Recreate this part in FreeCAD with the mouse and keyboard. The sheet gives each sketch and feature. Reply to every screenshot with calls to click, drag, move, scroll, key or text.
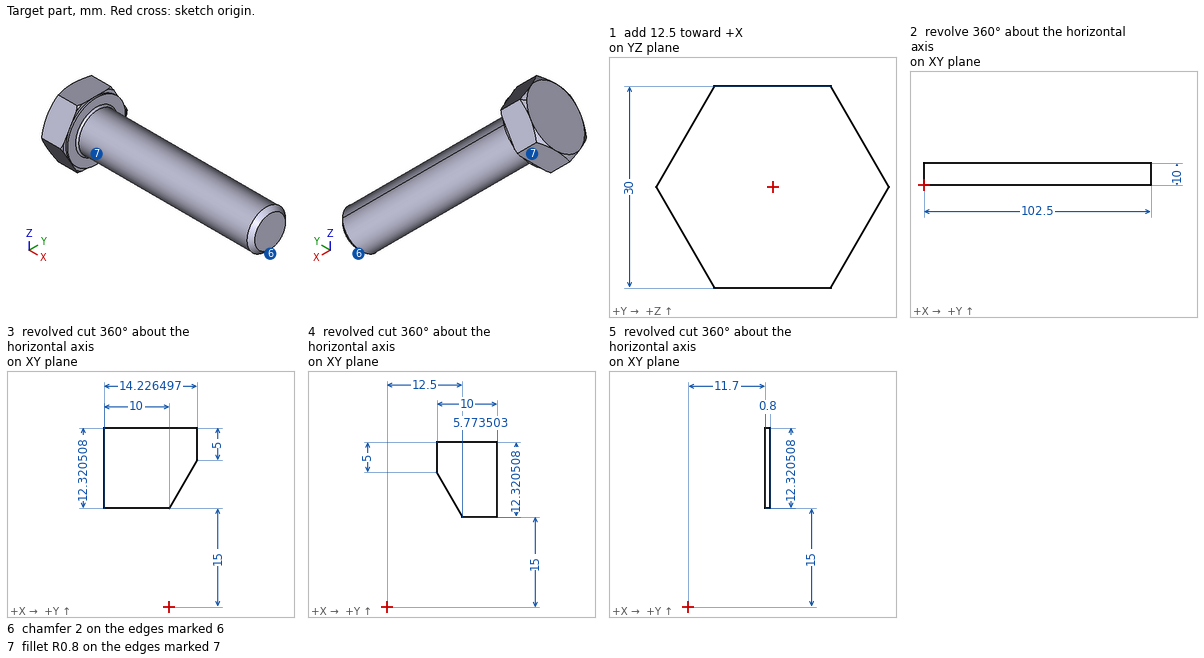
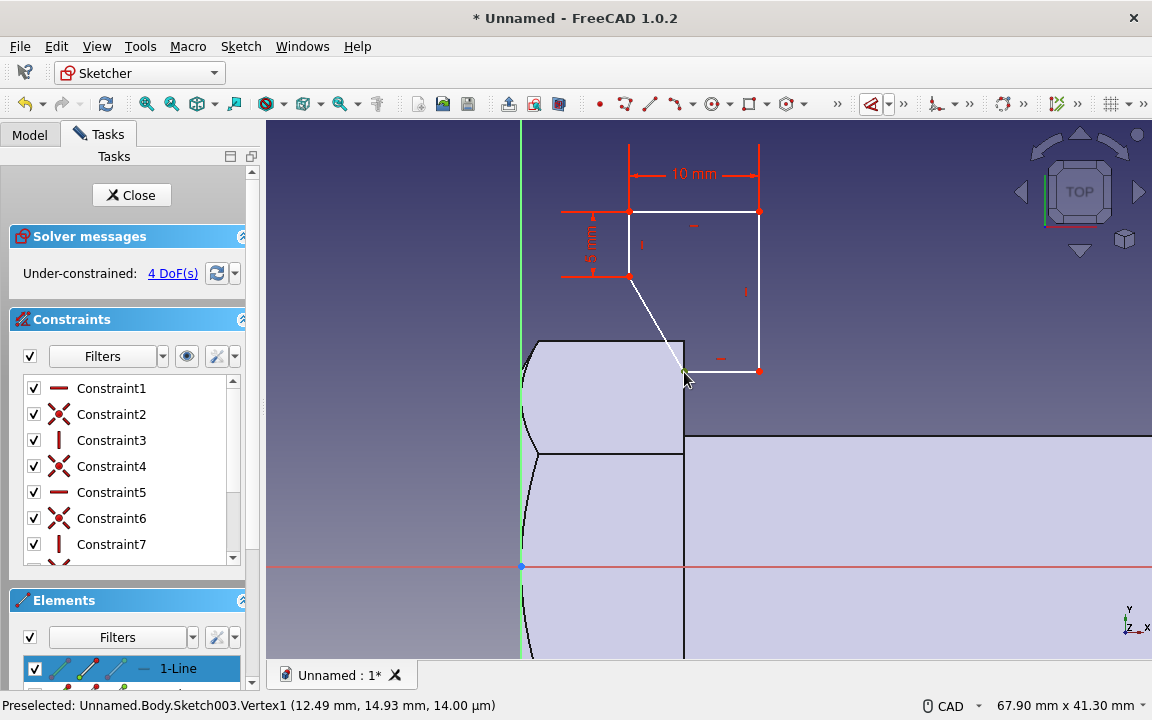
key(i)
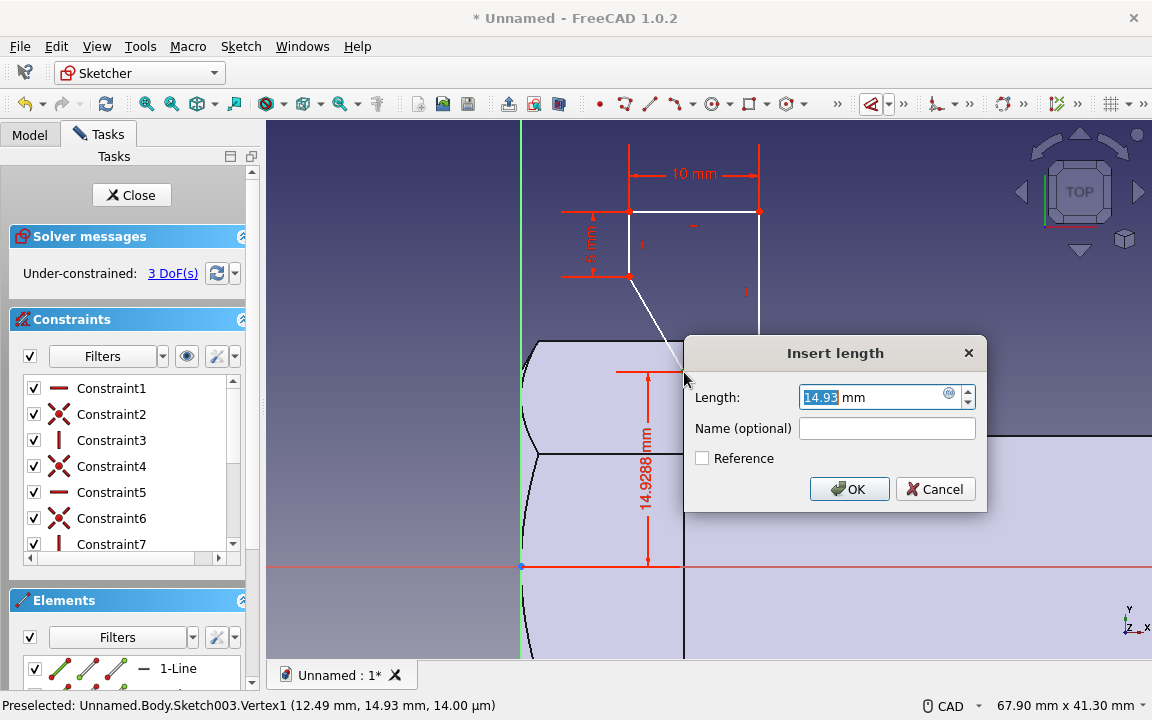
text(15)
key(Return)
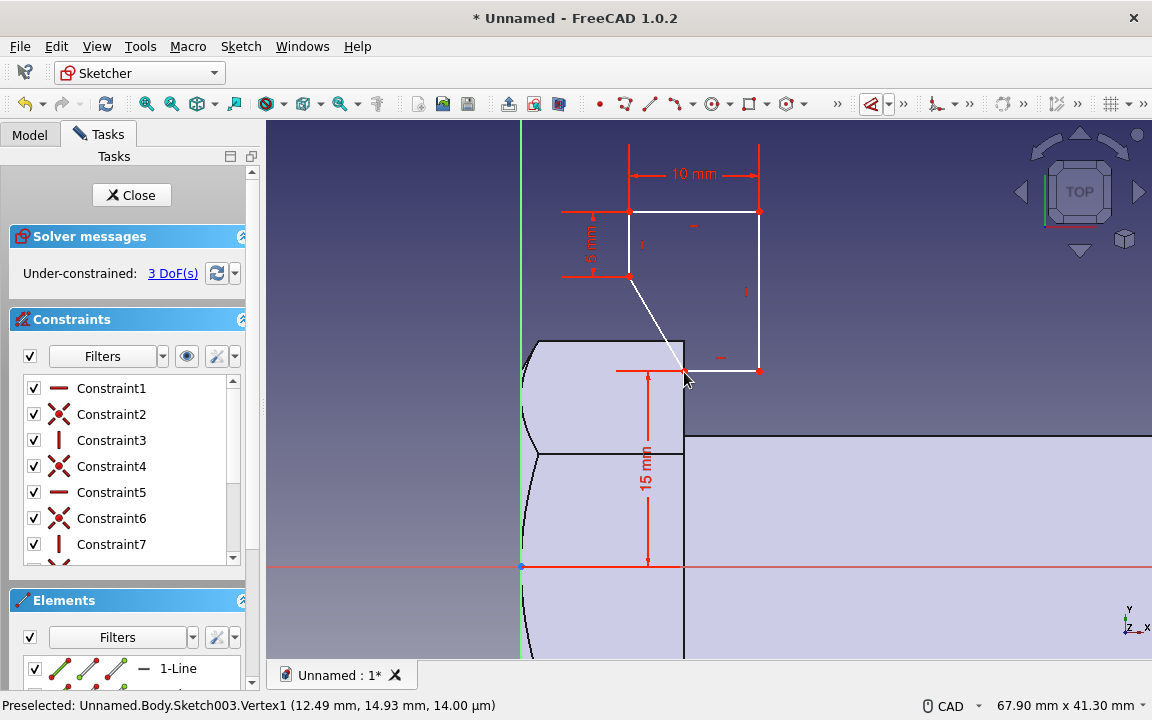
click(684, 371)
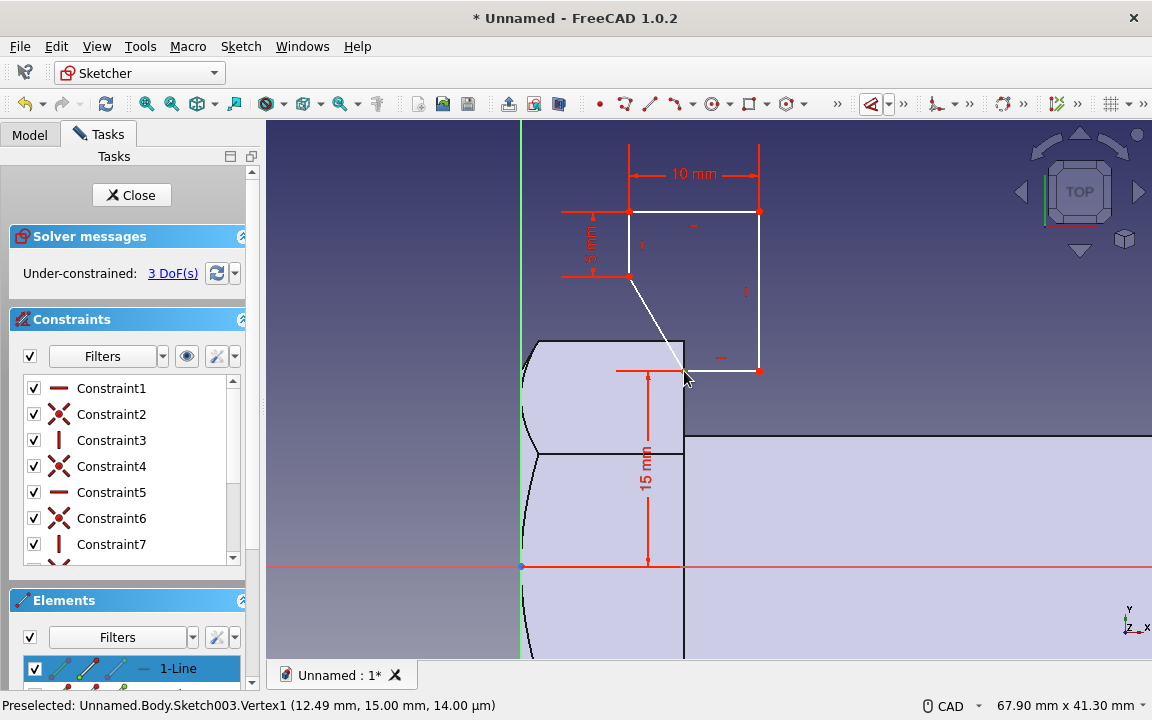
click(888, 104)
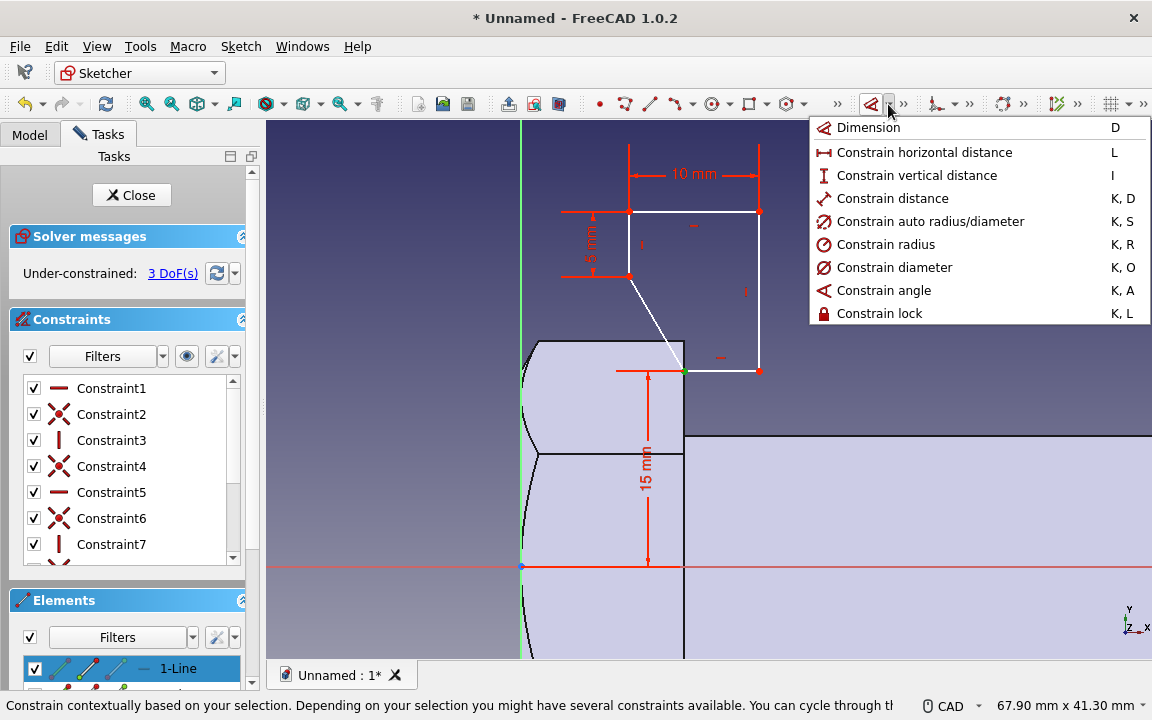
click(980, 152)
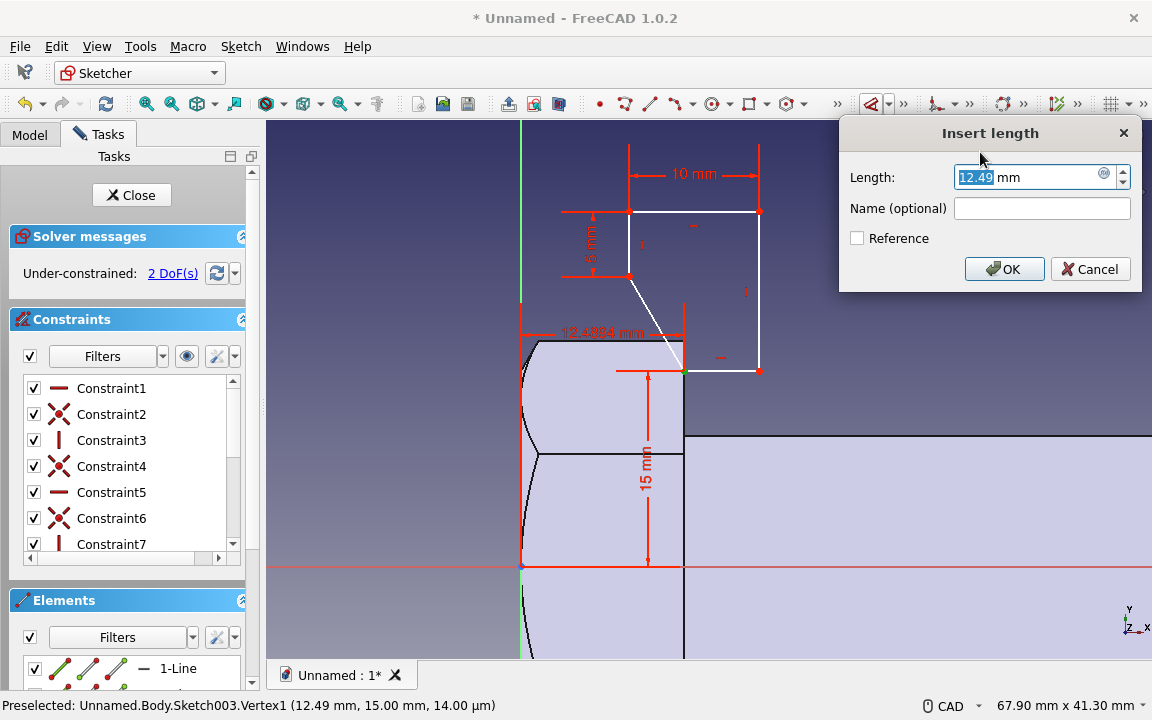
text(12.5)
key(Return)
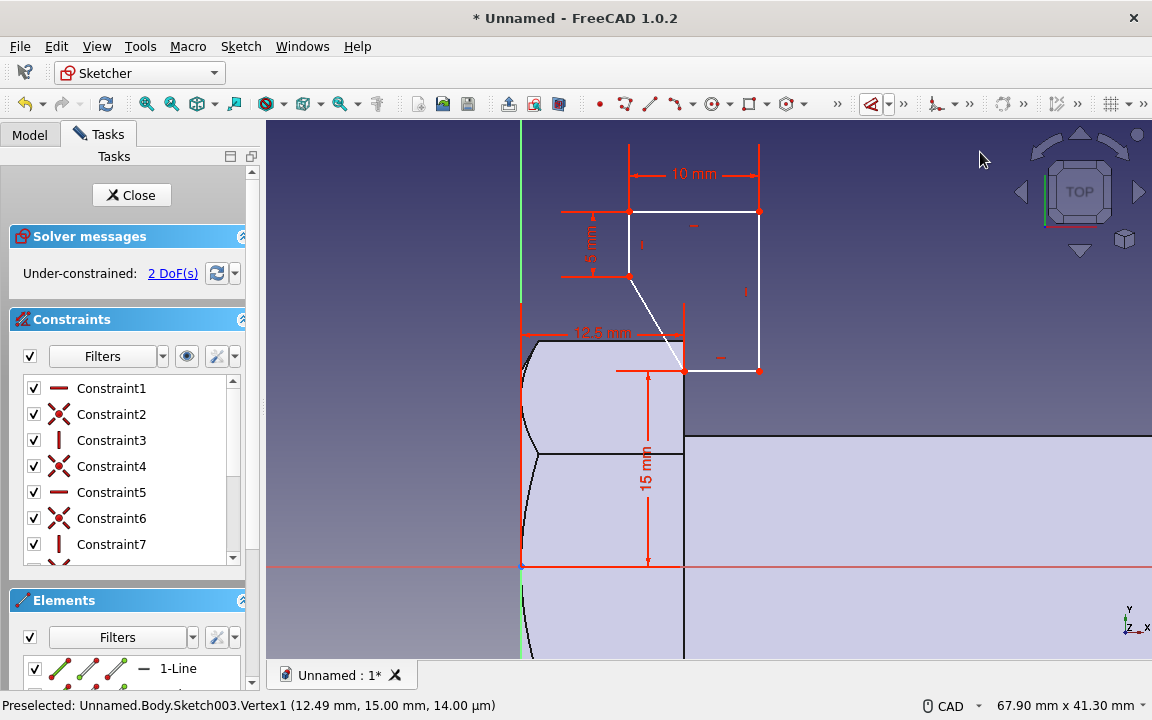
click(707, 371)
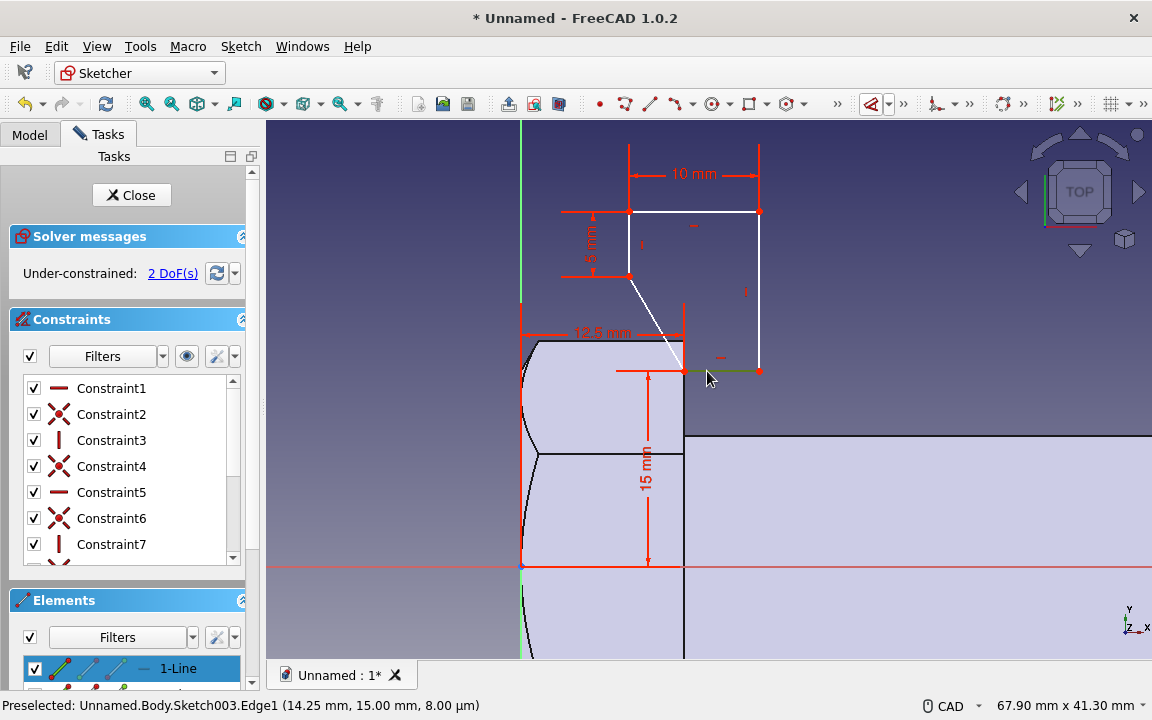
key(l)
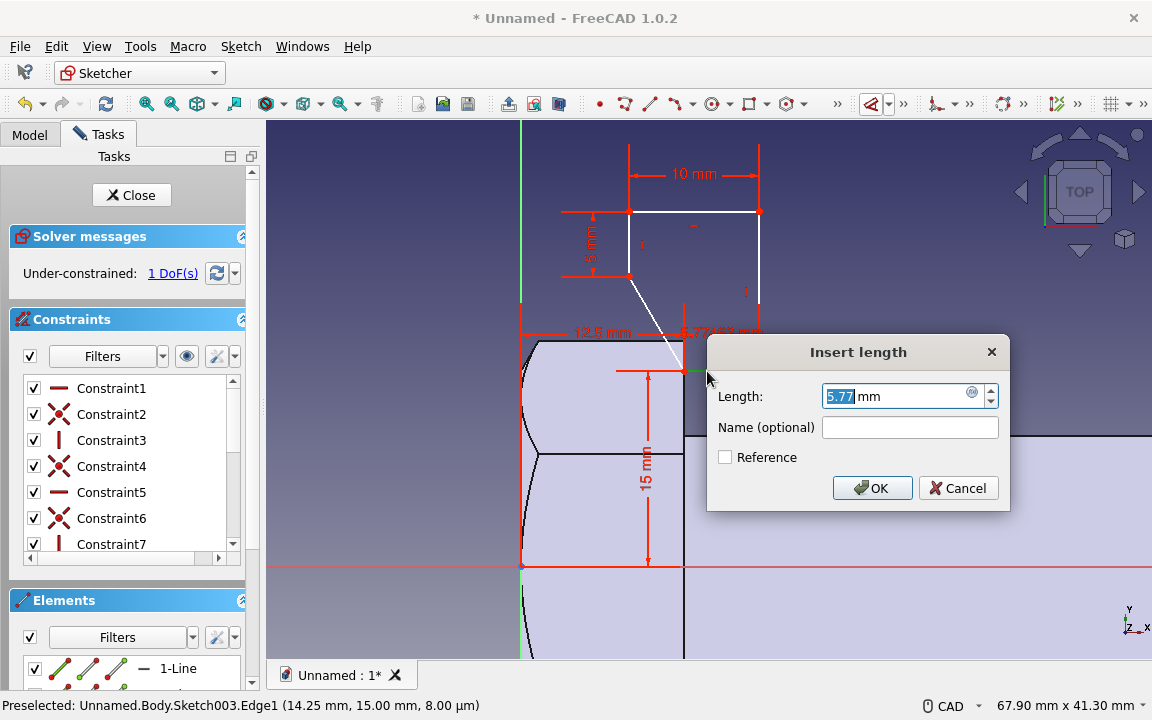
text(5.773503)
key(Return)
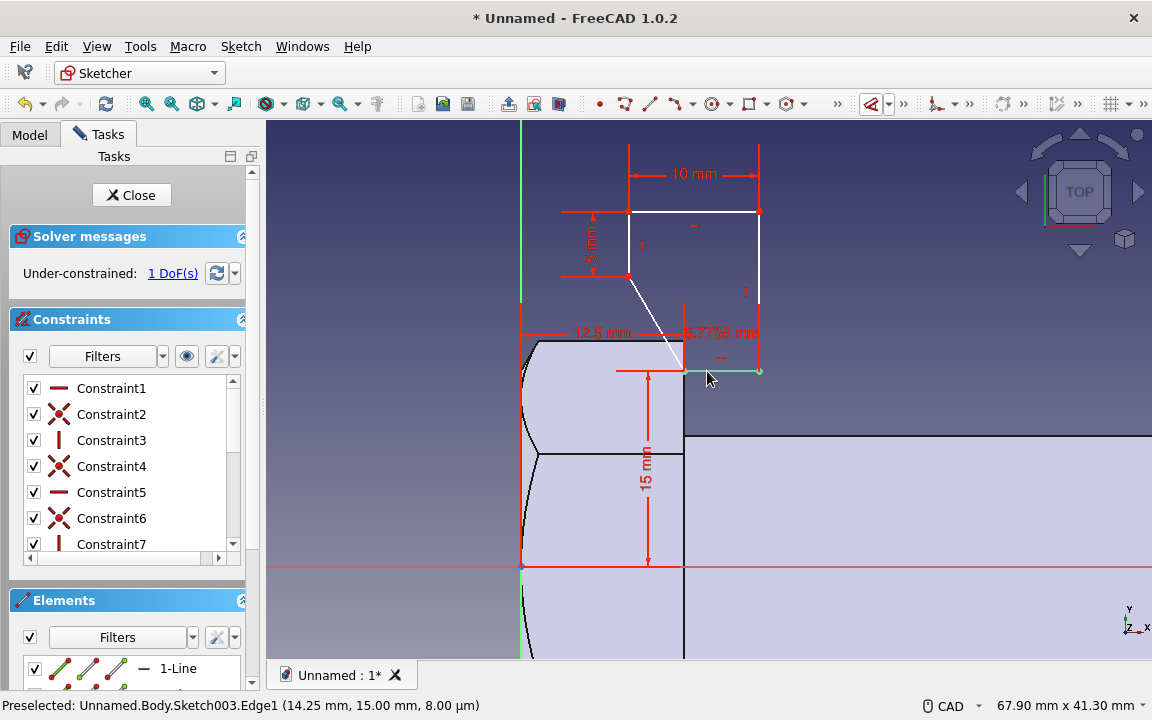
click(759, 323)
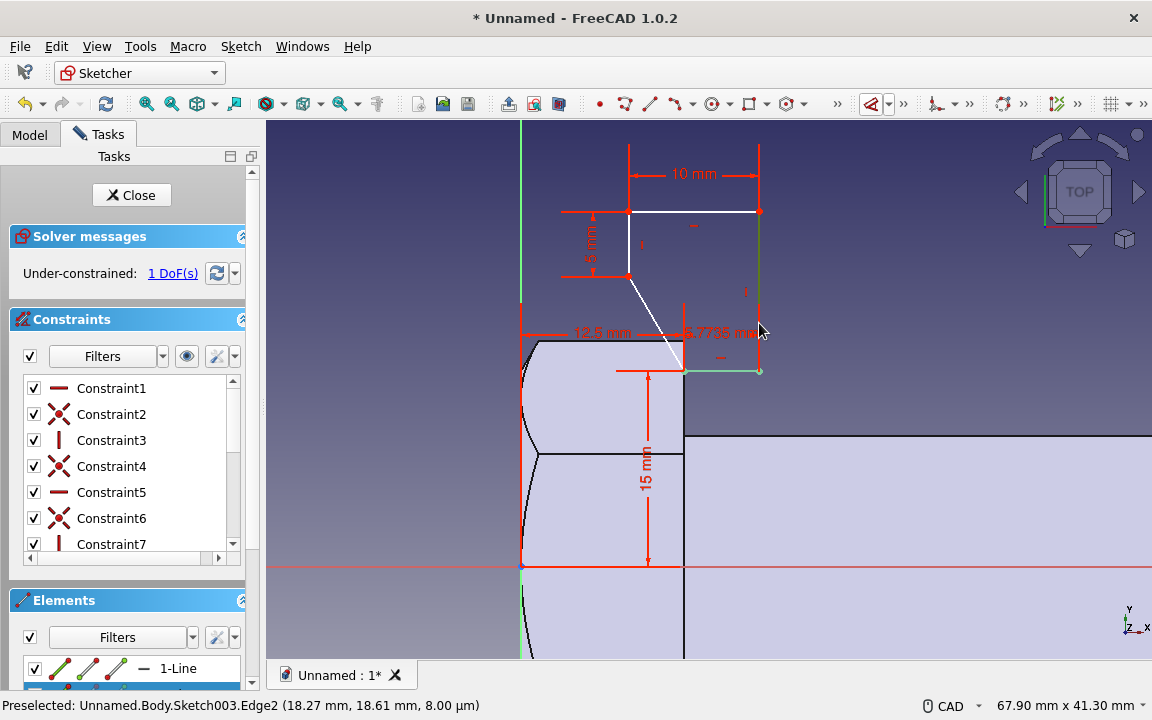
key(i)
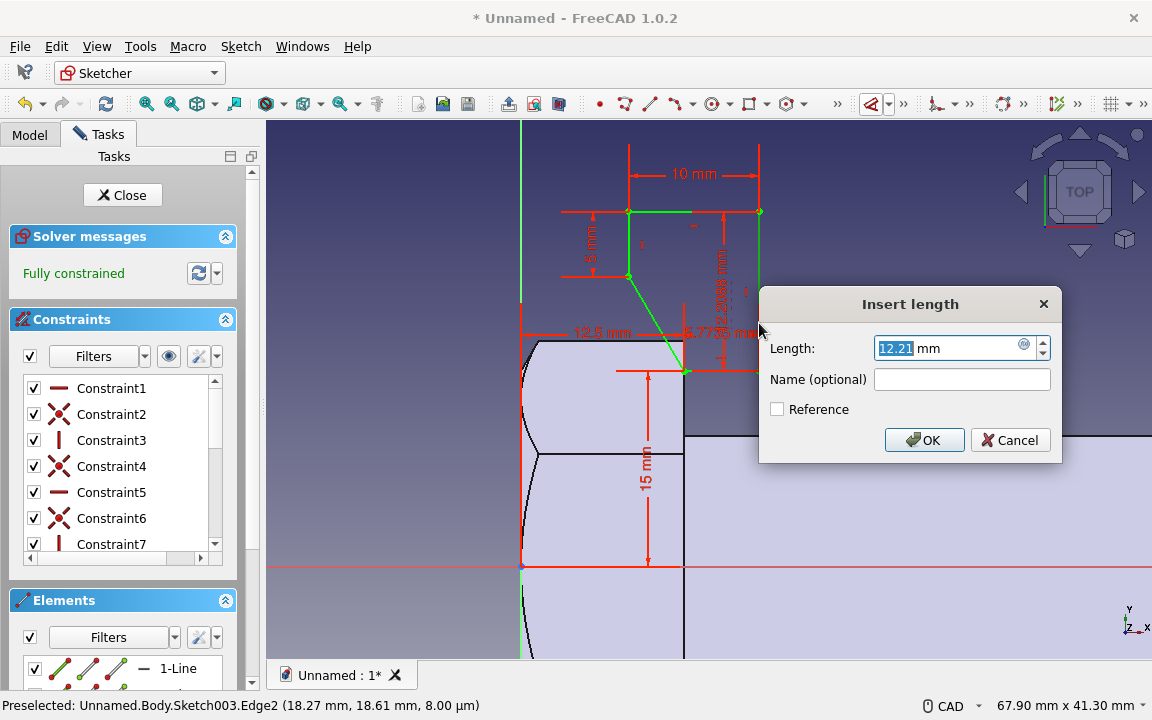
text(12.320508)
key(Return)